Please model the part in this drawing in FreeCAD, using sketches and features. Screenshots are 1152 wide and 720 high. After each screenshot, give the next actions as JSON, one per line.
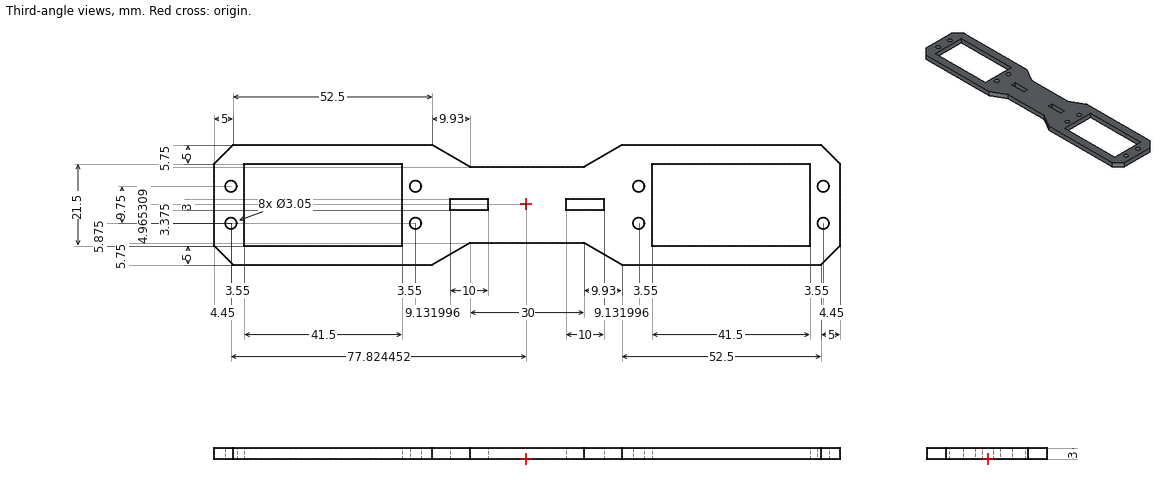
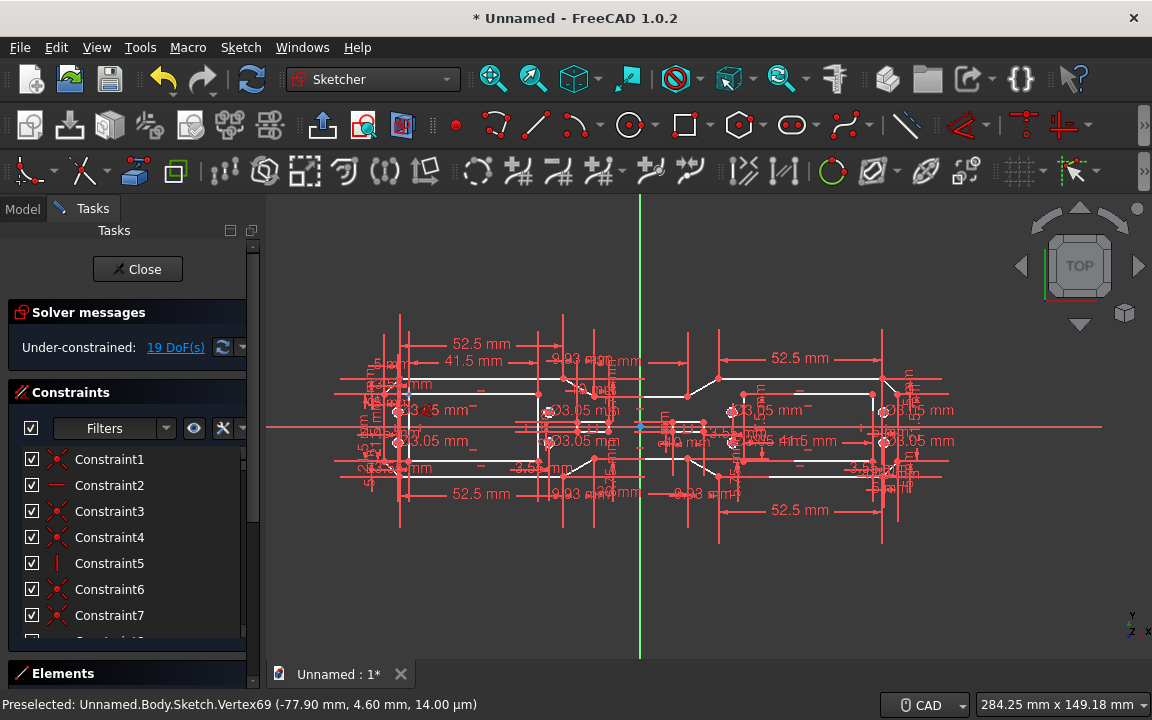
{"action": "scroll", "coordinate": [398, 443], "scroll_direction": "up", "scroll_amount": 2}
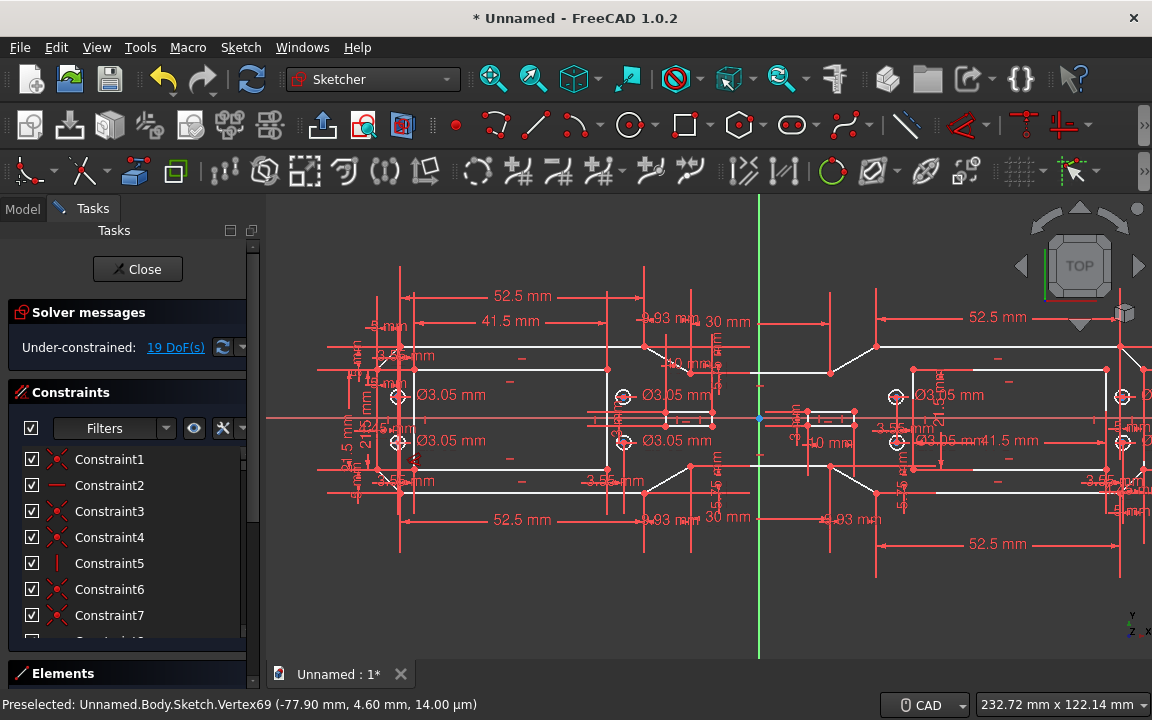
{"action": "left_click", "coordinate": [398, 443]}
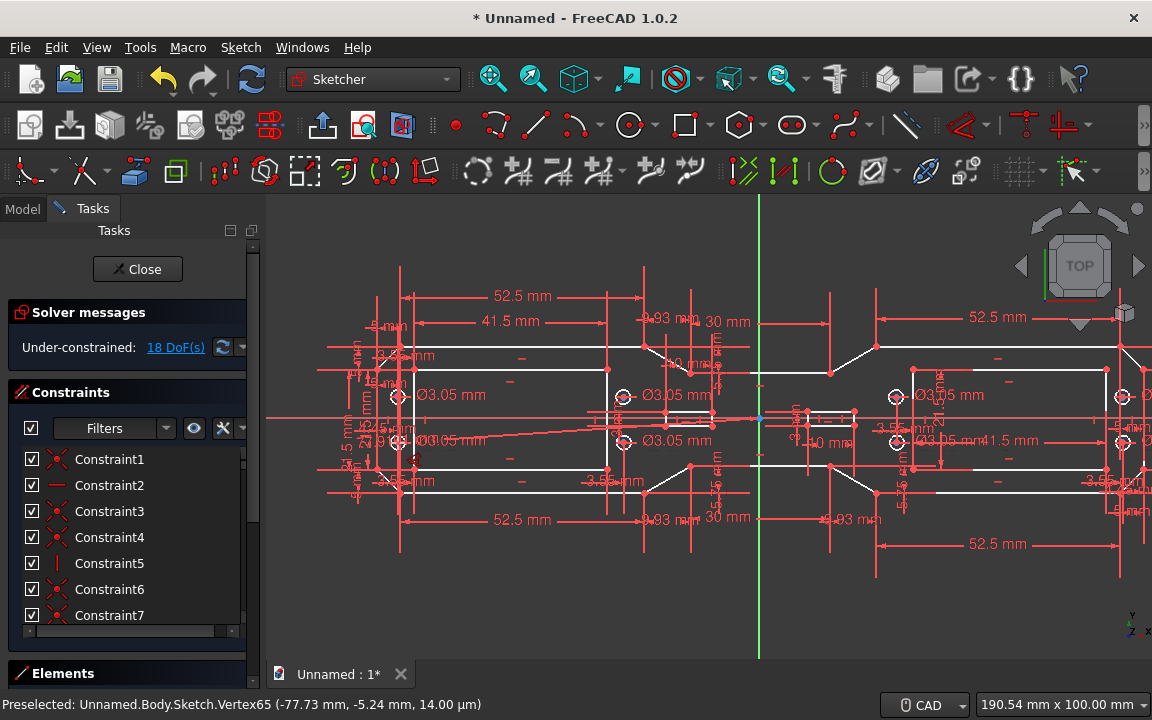
{"action": "left_click", "coordinate": [398, 397]}
{"action": "left_click", "coordinate": [316, 404]}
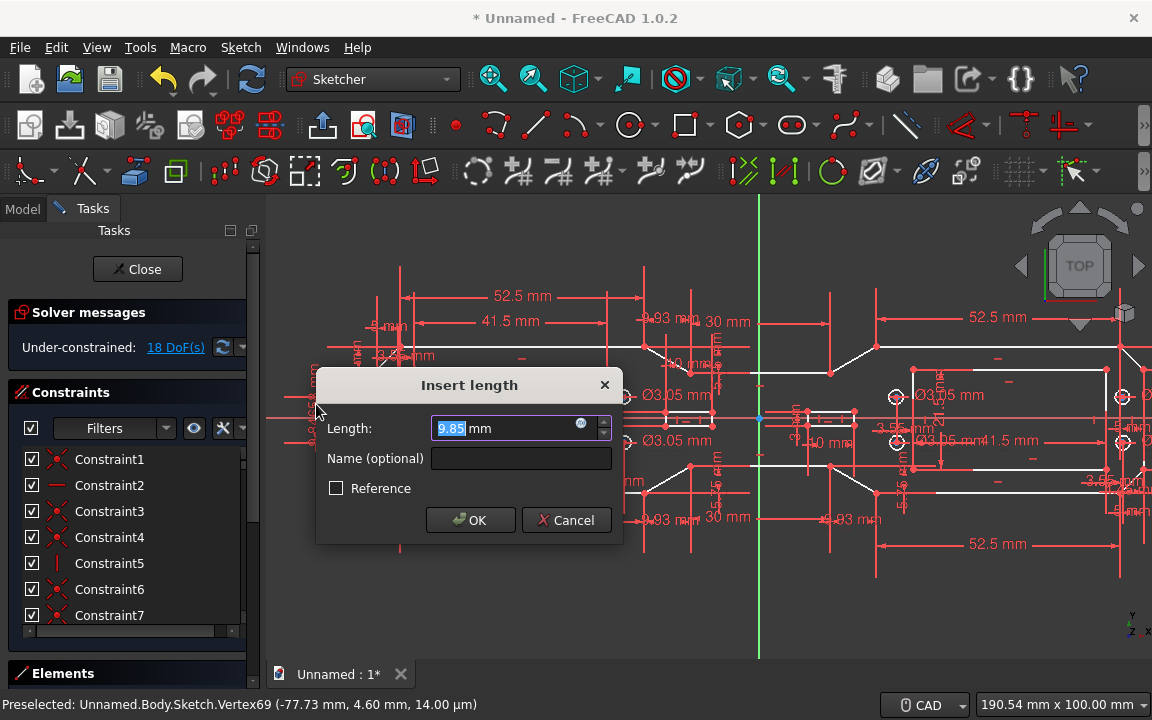
{"action": "type", "text": "9.75"}
{"action": "key", "text": "Return"}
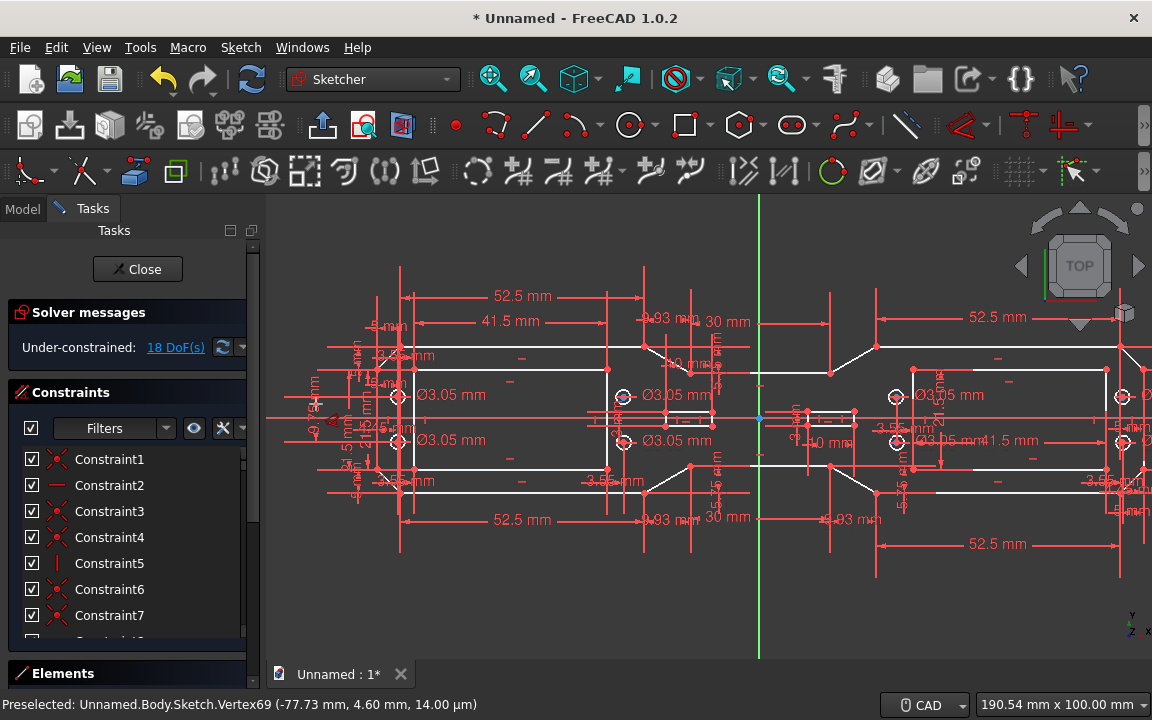
{"action": "scroll", "coordinate": [607, 370], "scroll_direction": "up", "scroll_amount": 5}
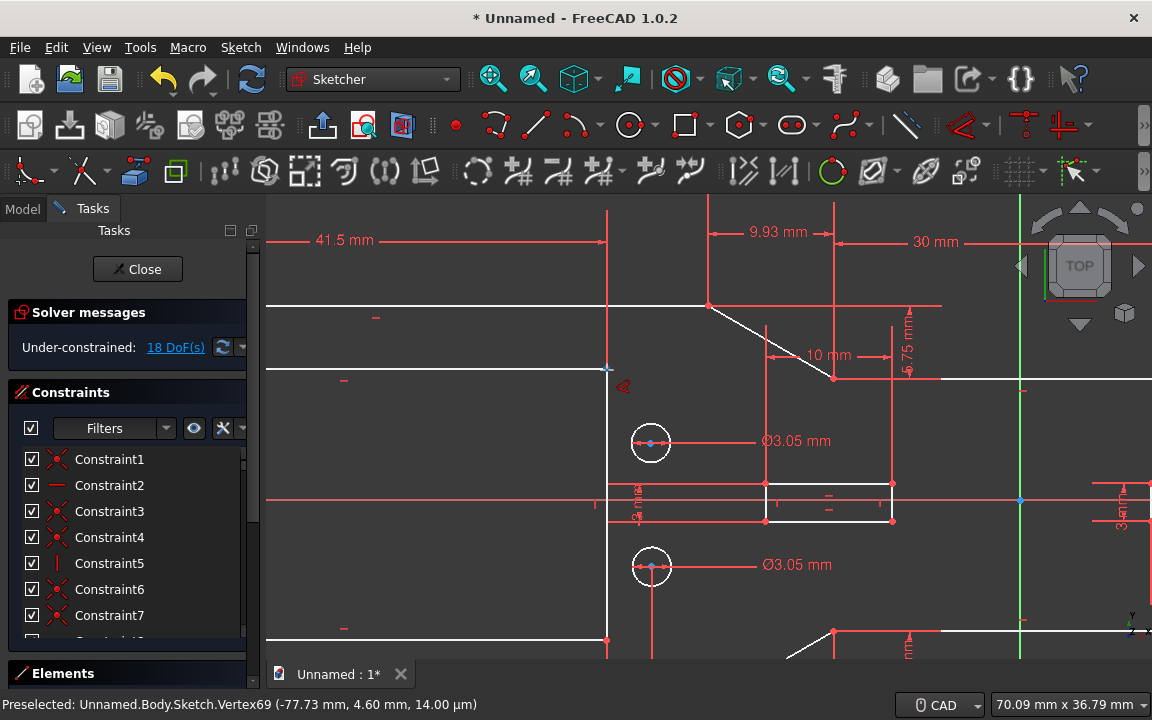
{"action": "left_click", "coordinate": [607, 369]}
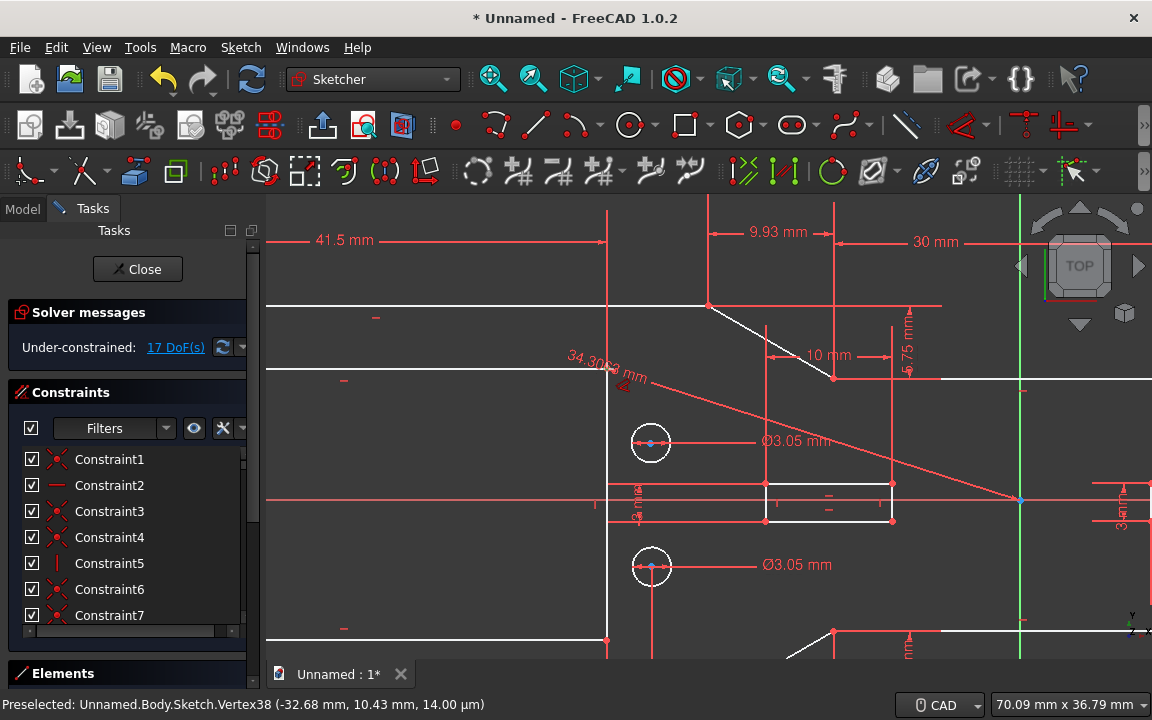
{"action": "left_click", "coordinate": [651, 443]}
{"action": "left_click", "coordinate": [629, 335]}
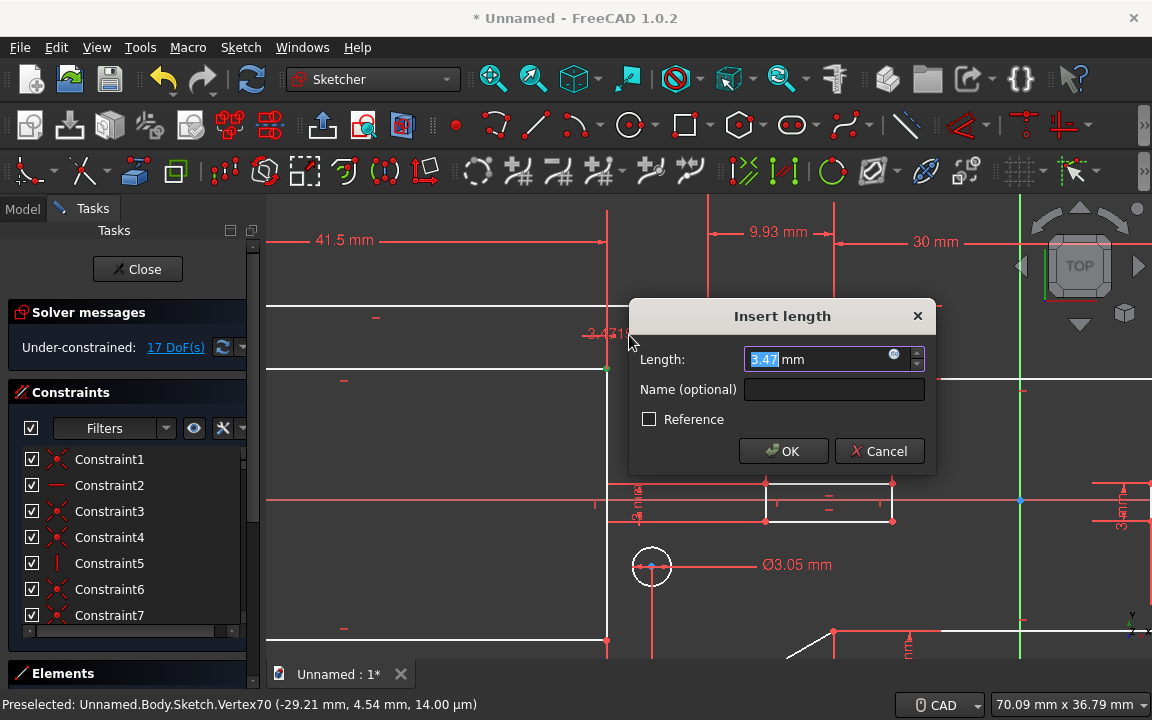
{"action": "type", "text": "3.55"}
{"action": "key", "text": "Return"}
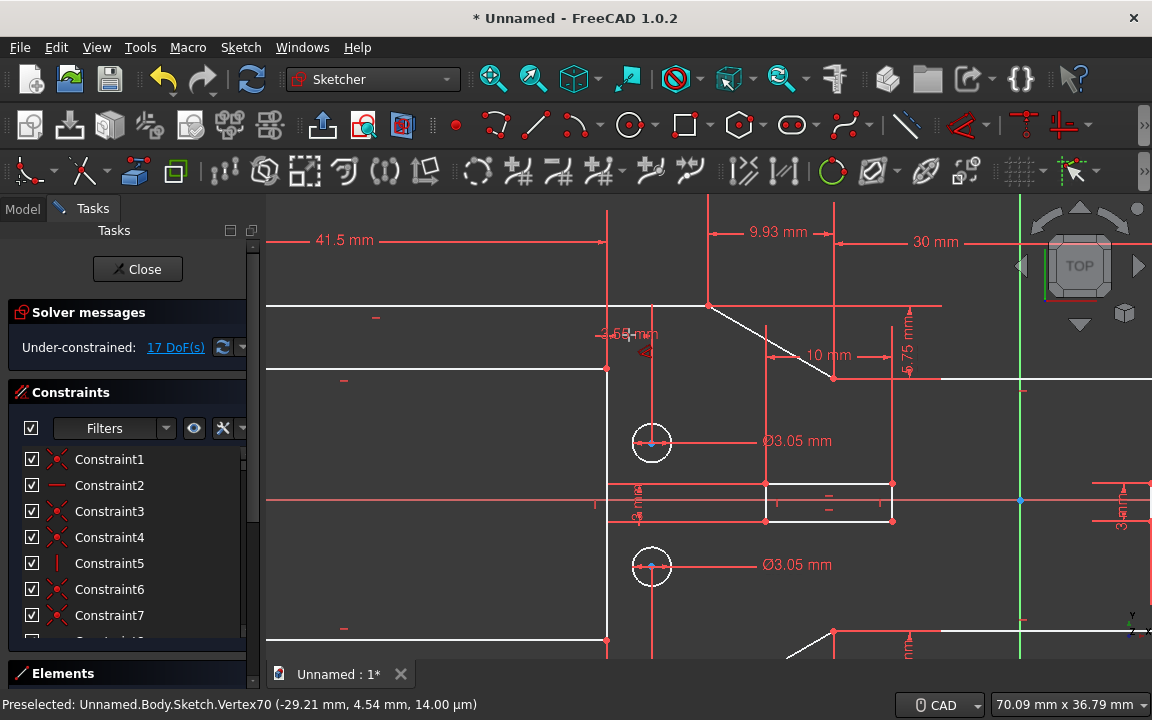
{"action": "scroll", "coordinate": [516, 402], "scroll_direction": "down", "scroll_amount": 7}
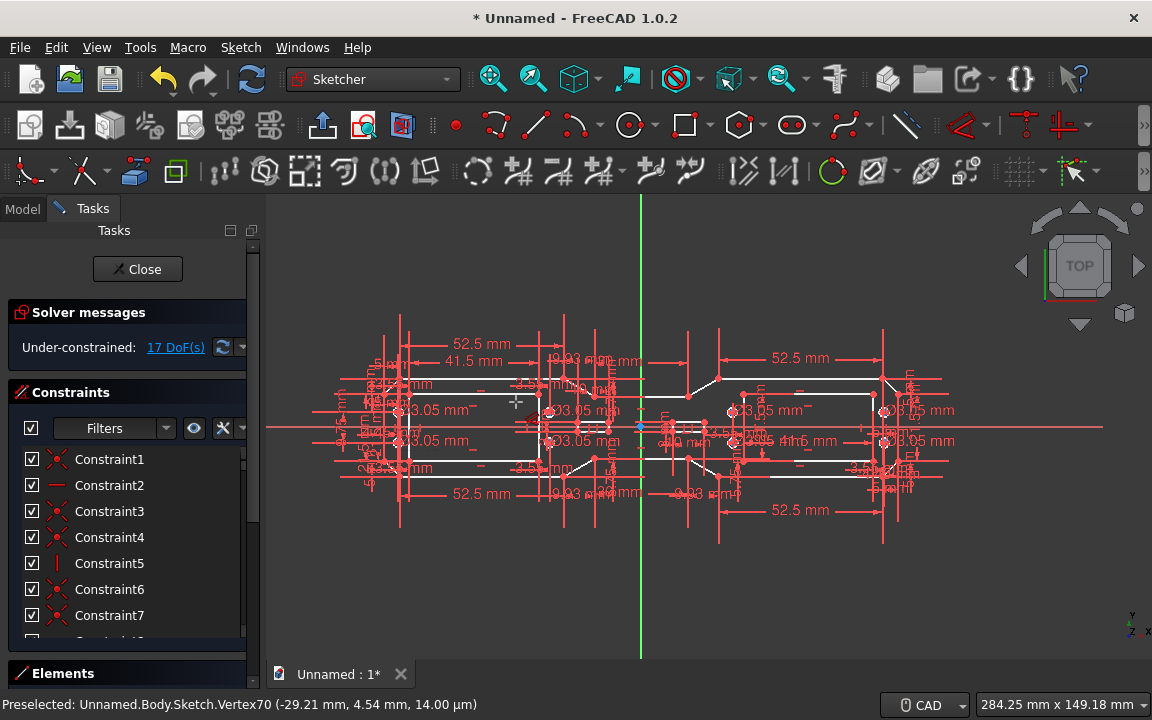
{"action": "scroll", "coordinate": [550, 443], "scroll_direction": "up", "scroll_amount": 2}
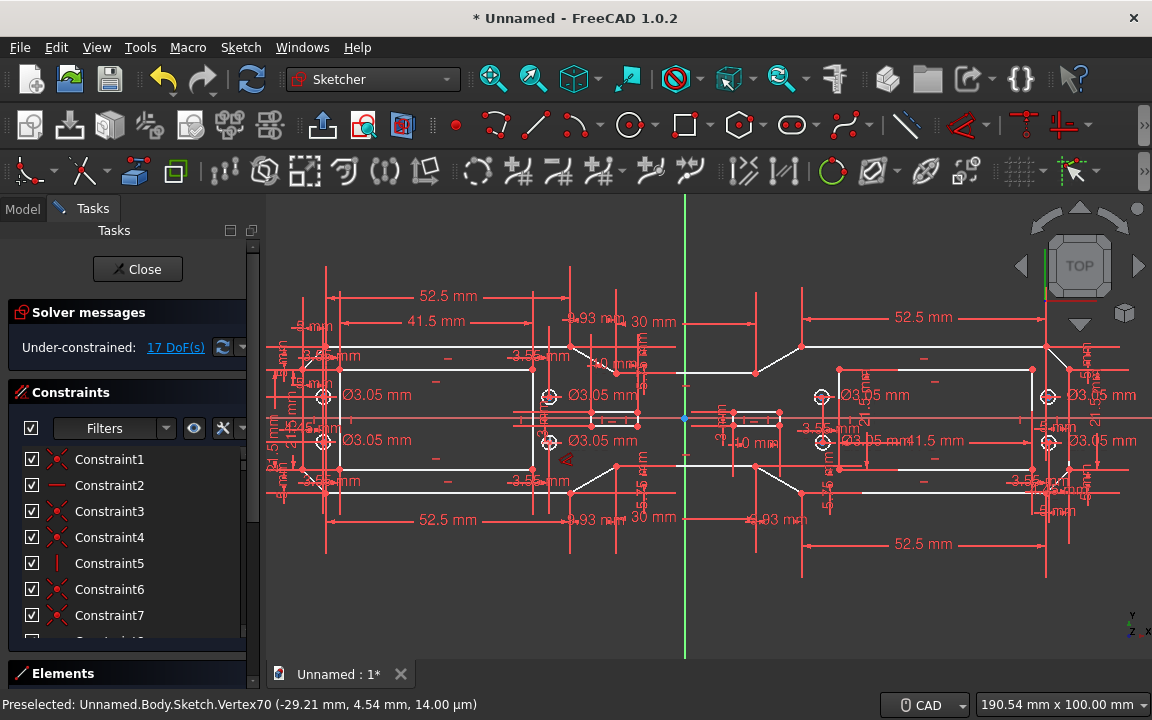
{"action": "left_click", "coordinate": [549, 443]}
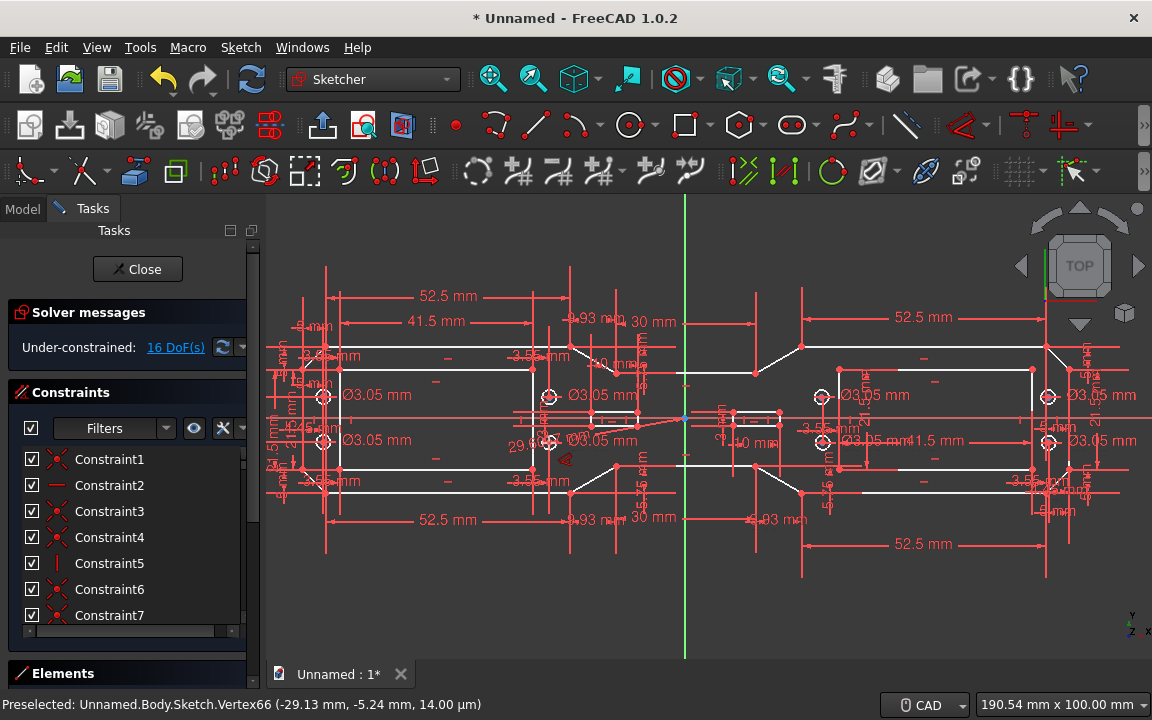
{"action": "left_click", "coordinate": [549, 397]}
{"action": "left_click", "coordinate": [515, 404]}